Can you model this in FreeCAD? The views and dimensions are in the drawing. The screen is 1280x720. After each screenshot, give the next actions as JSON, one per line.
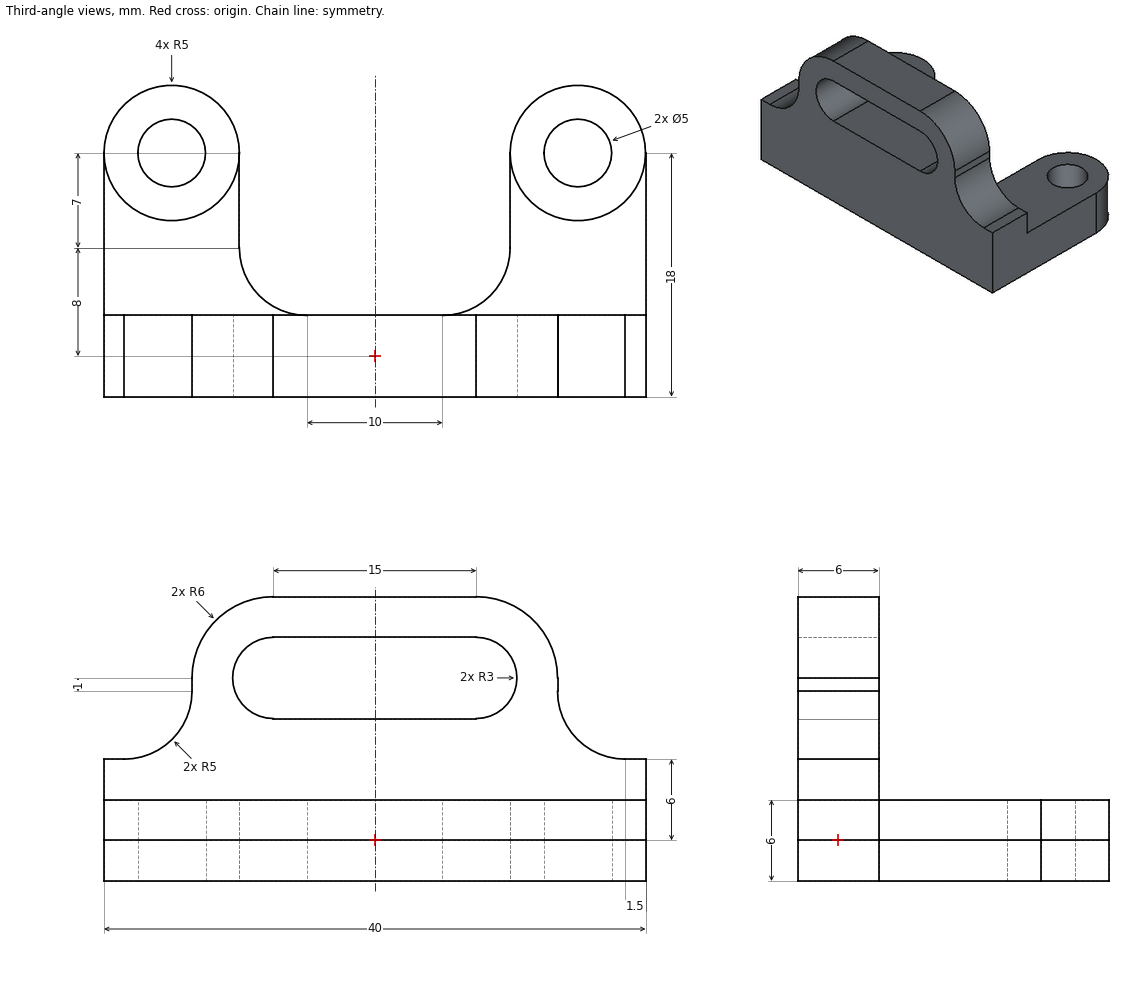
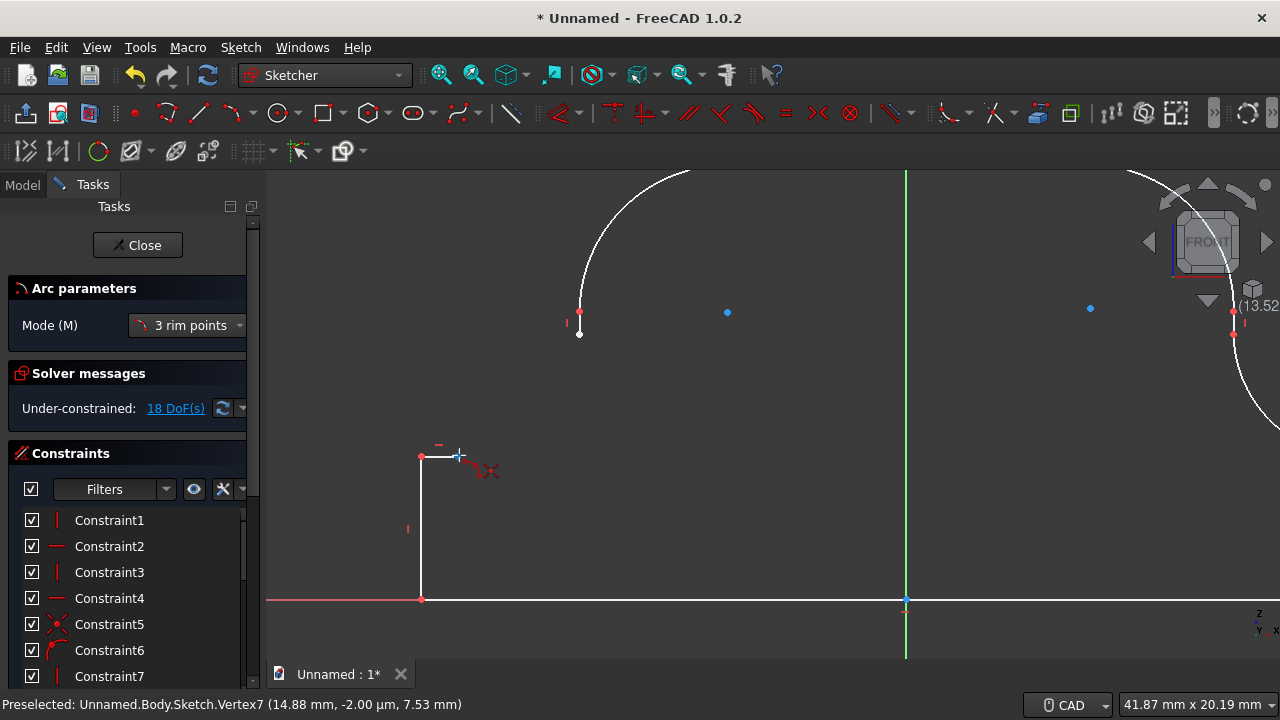
{"action": "left_click", "coordinate": [458, 457]}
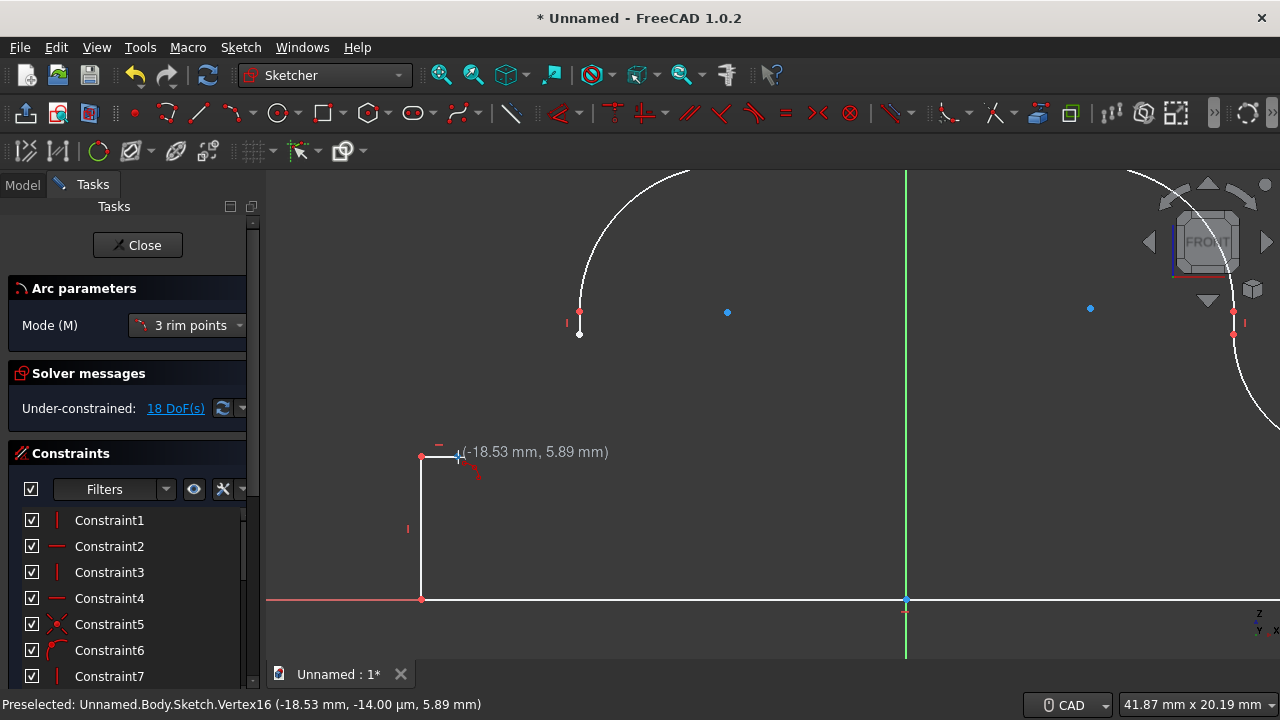
{"action": "scroll", "coordinate": [579, 333], "scroll_direction": "up", "scroll_amount": 2}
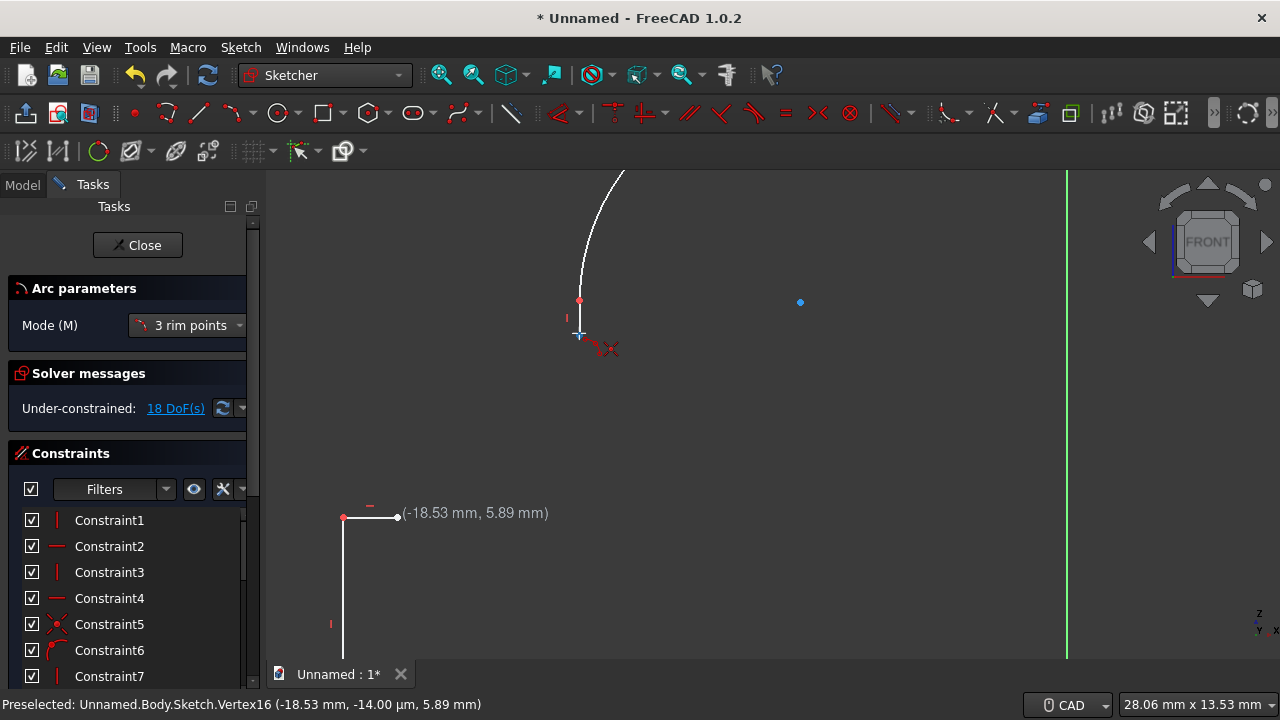
{"action": "left_click", "coordinate": [580, 335]}
{"action": "left_click", "coordinate": [527, 461]}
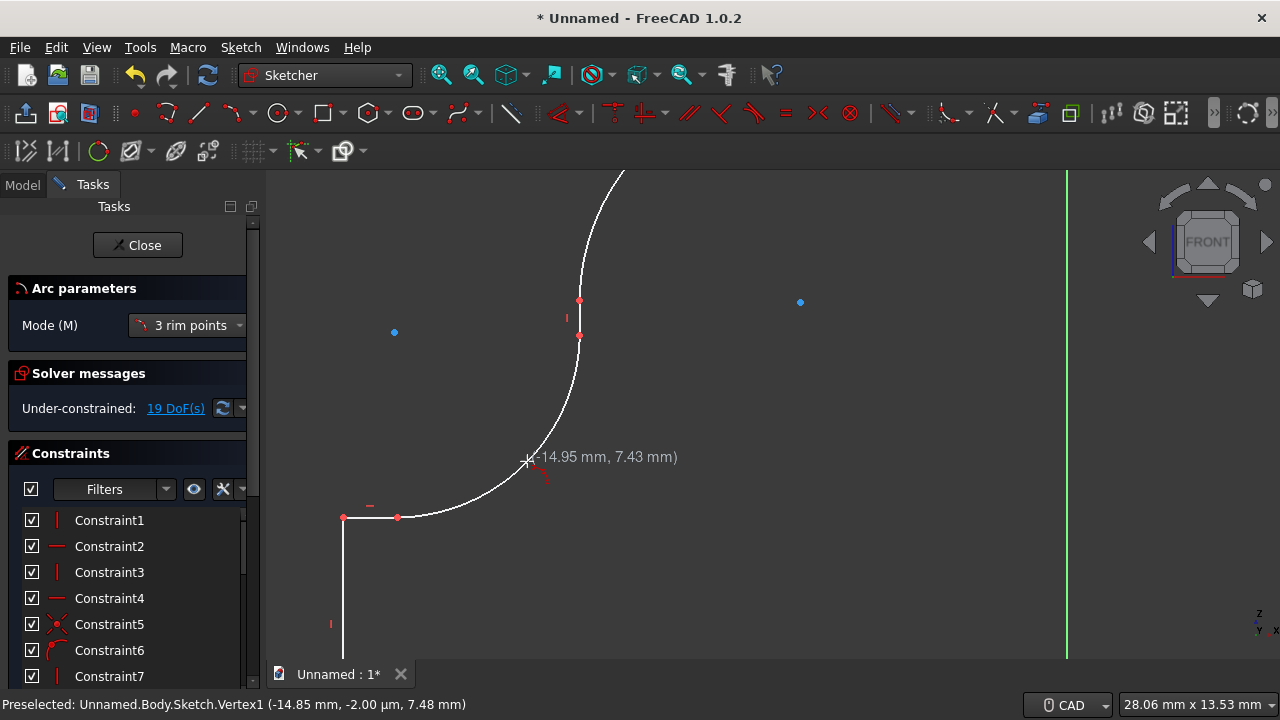
{"action": "left_click", "coordinate": [414, 114]}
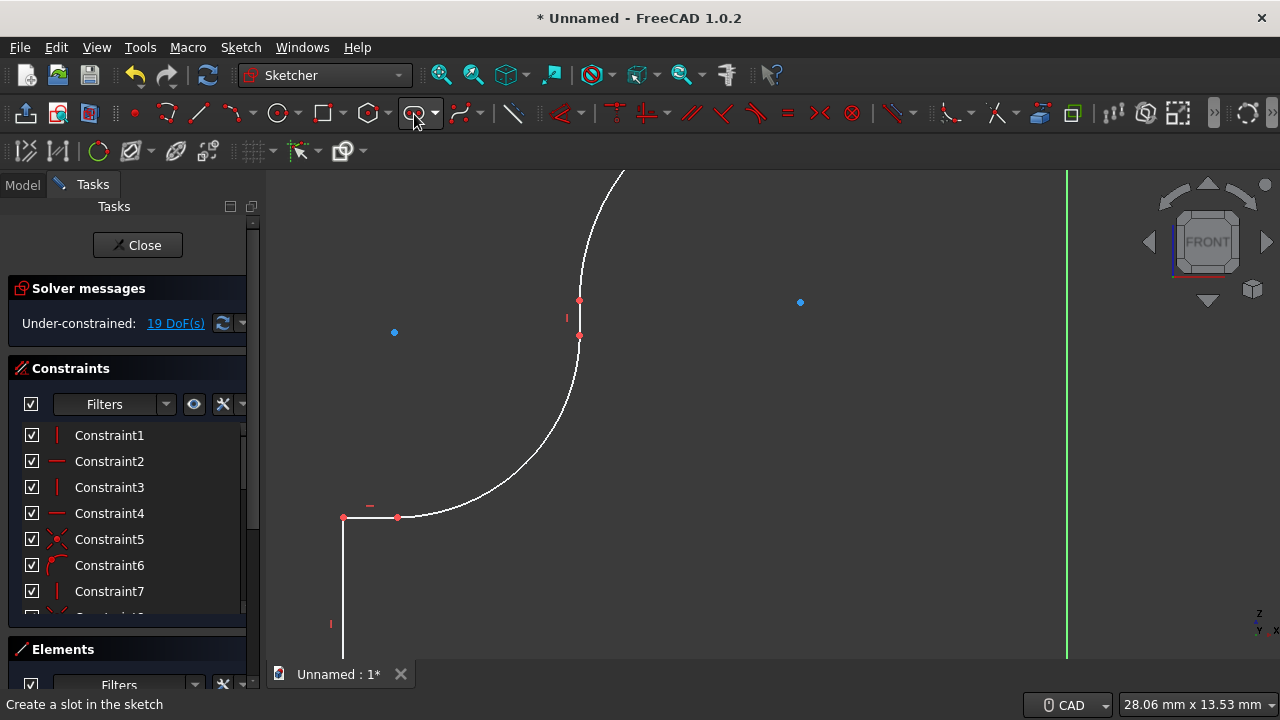
{"action": "left_click", "coordinate": [796, 297]}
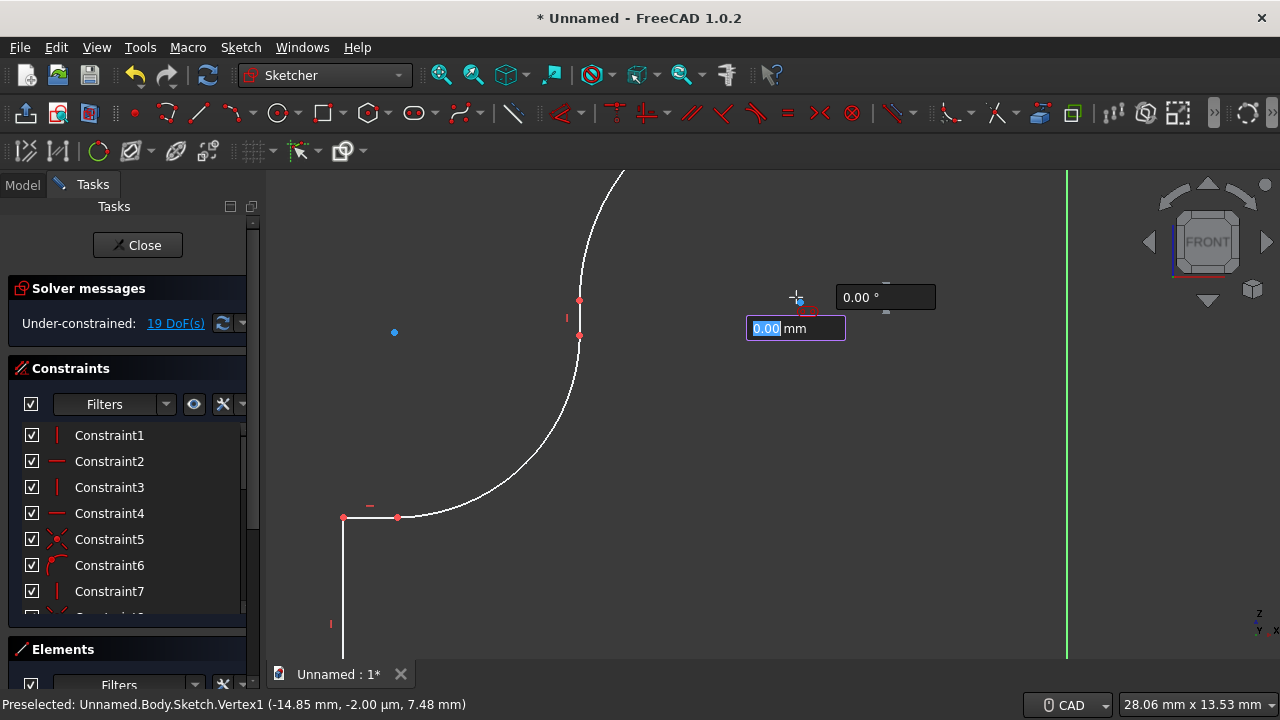
{"action": "scroll", "coordinate": [493, 420], "scroll_direction": "down", "scroll_amount": 5}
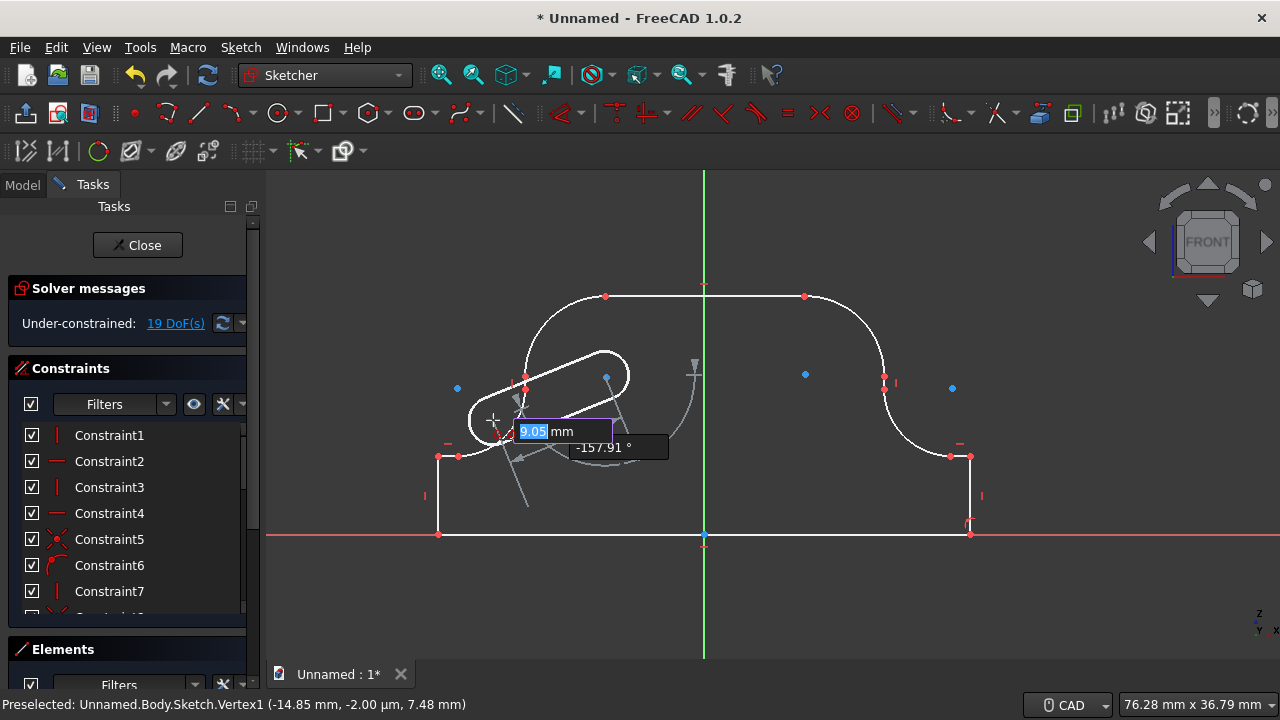
{"action": "left_click", "coordinate": [804, 375]}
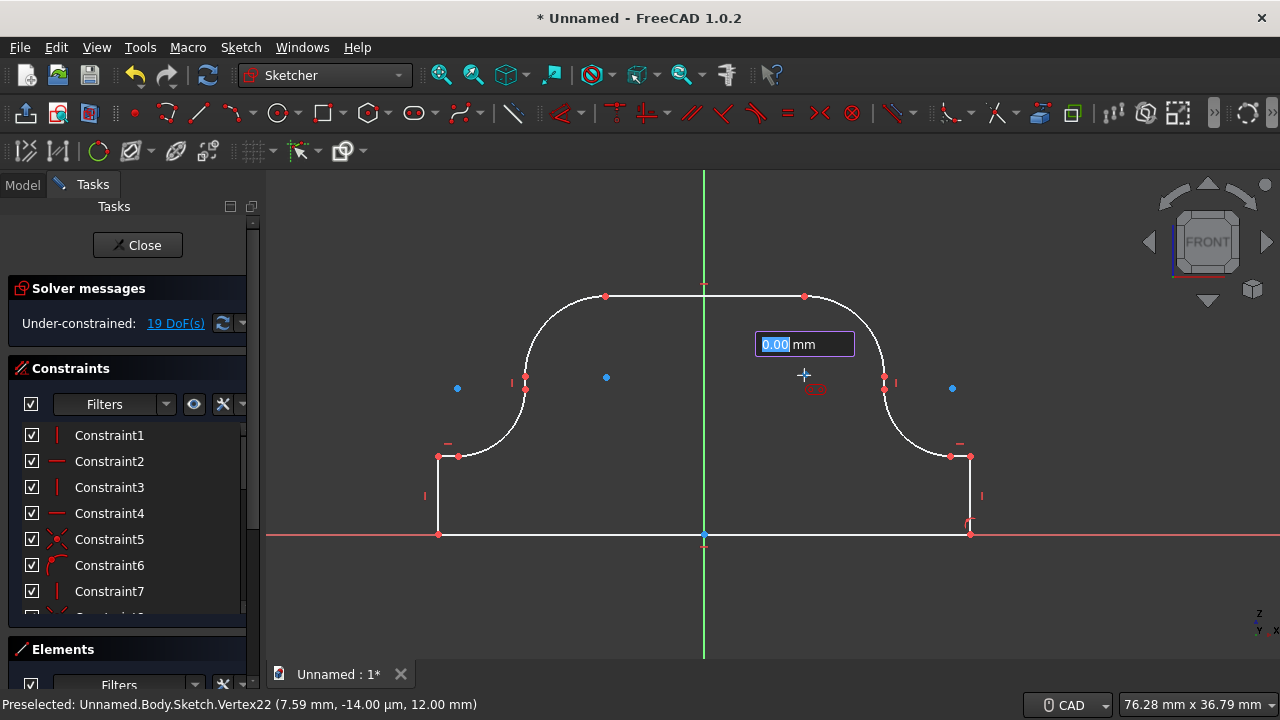
{"action": "left_click", "coordinate": [674, 415]}
{"action": "key", "text": "Escape"}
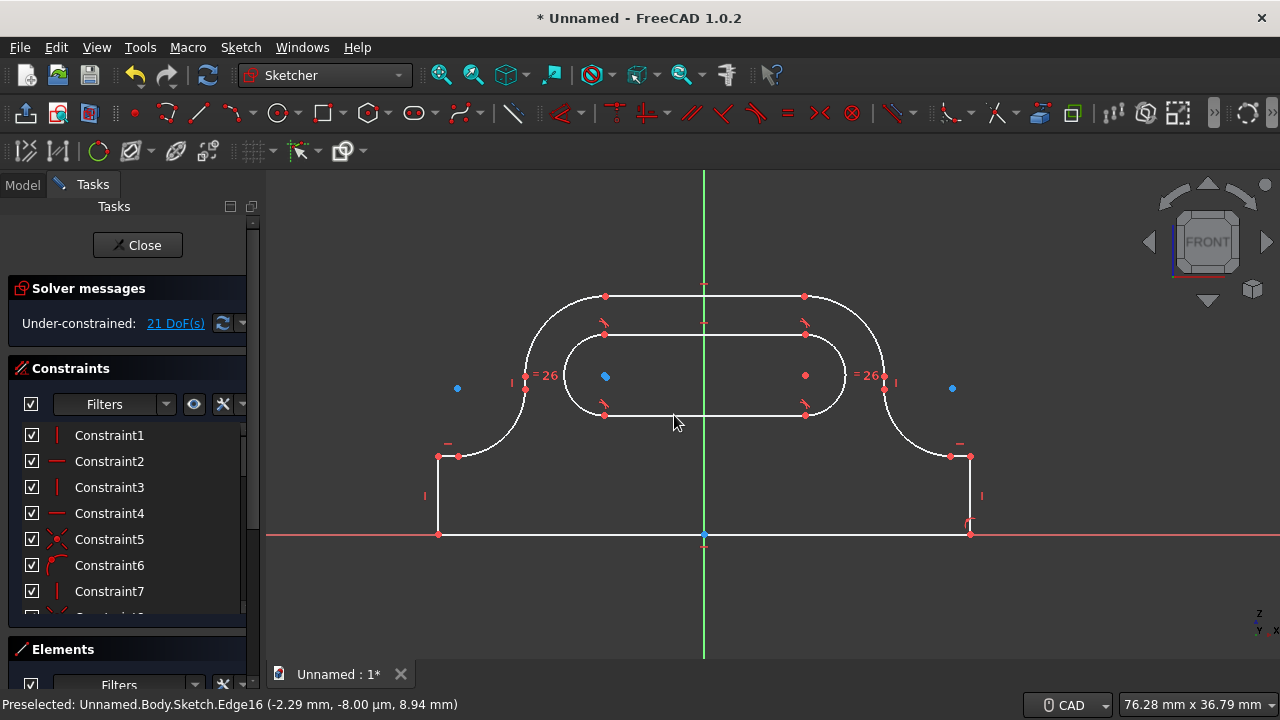
{"action": "scroll", "coordinate": [525, 383], "scroll_direction": "up", "scroll_amount": 4}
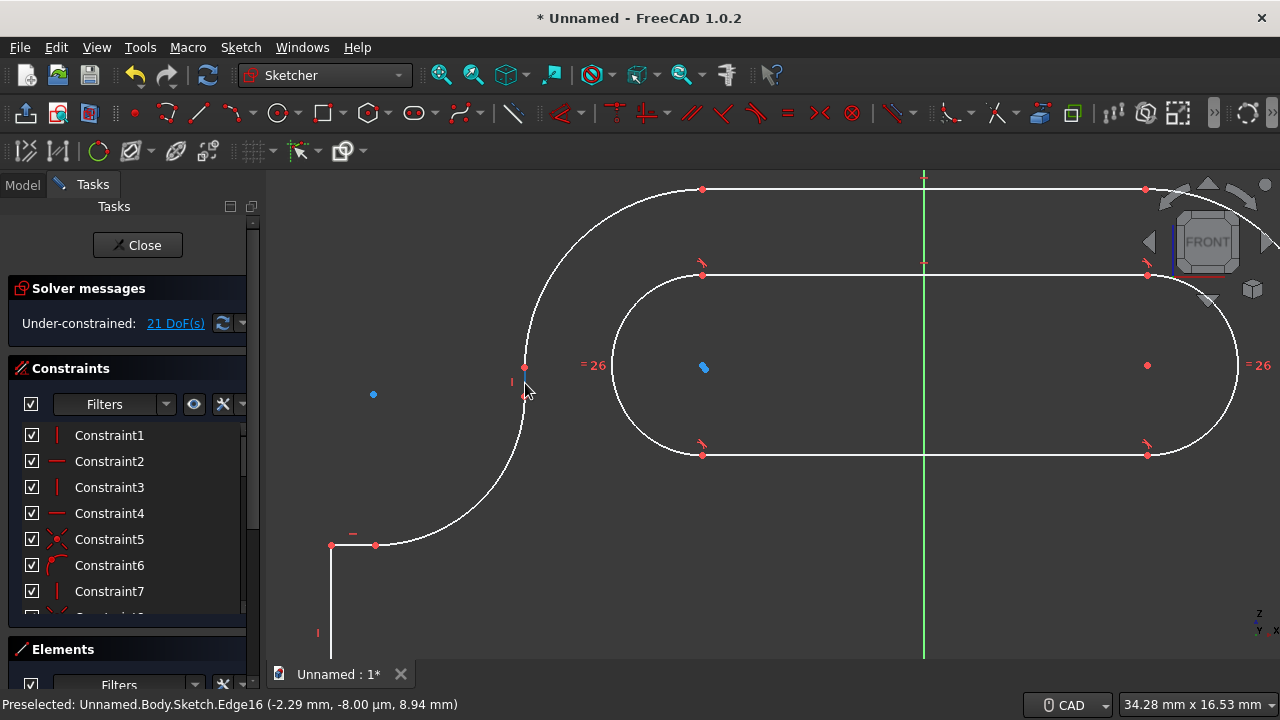
{"action": "left_click", "coordinate": [525, 382]}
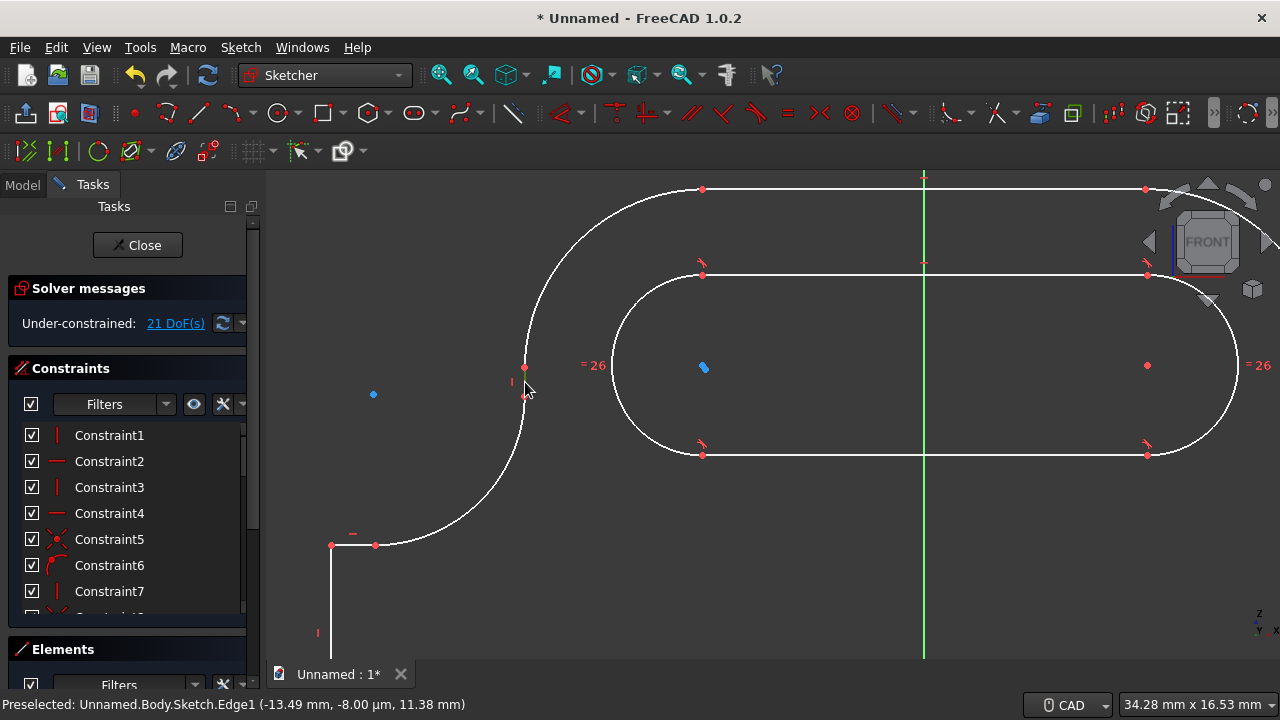
{"action": "left_click", "coordinate": [622, 209]}